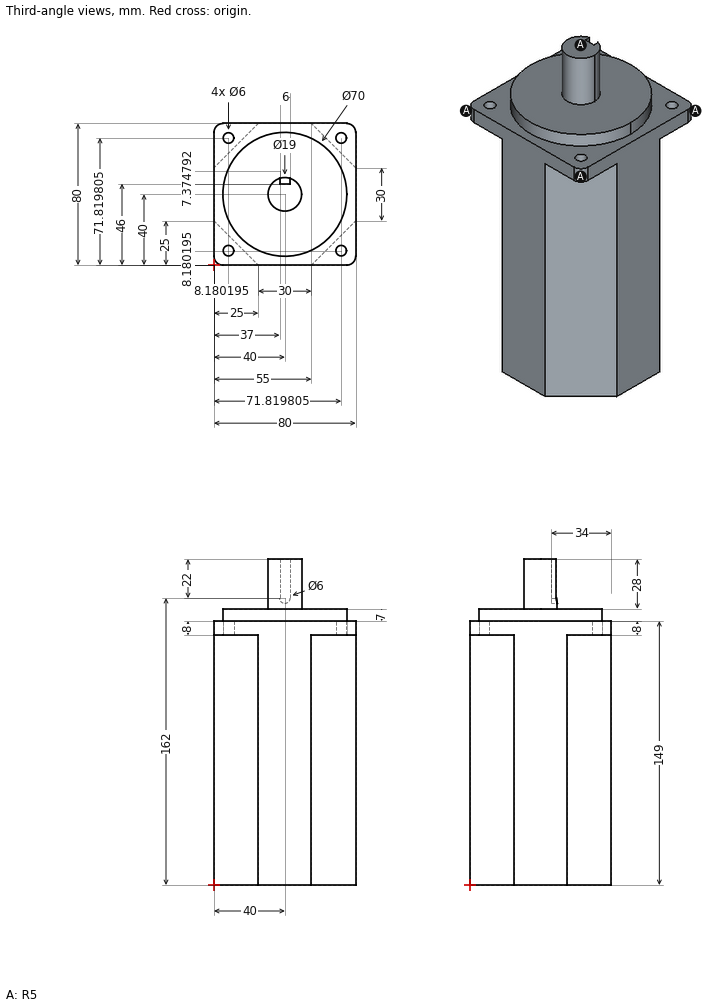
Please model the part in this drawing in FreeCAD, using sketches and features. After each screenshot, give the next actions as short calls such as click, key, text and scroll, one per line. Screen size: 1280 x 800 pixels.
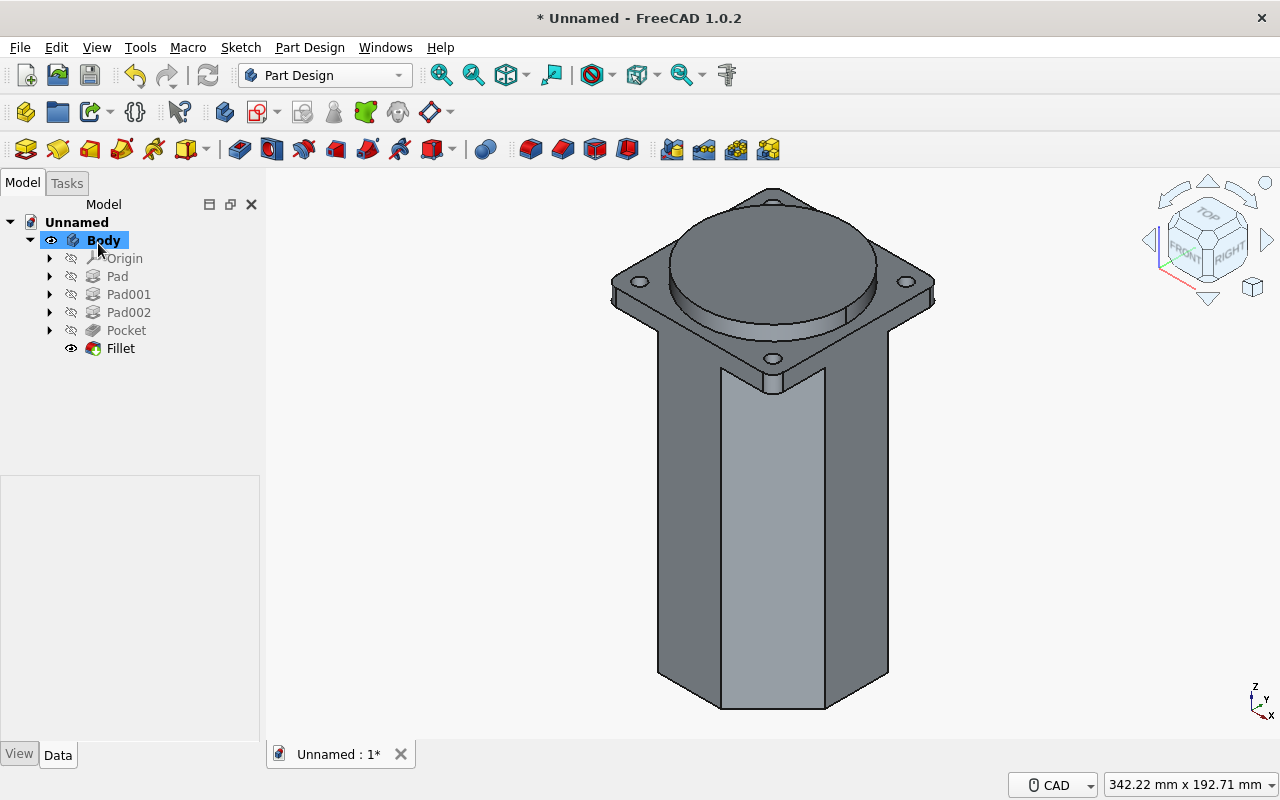
click(442, 76)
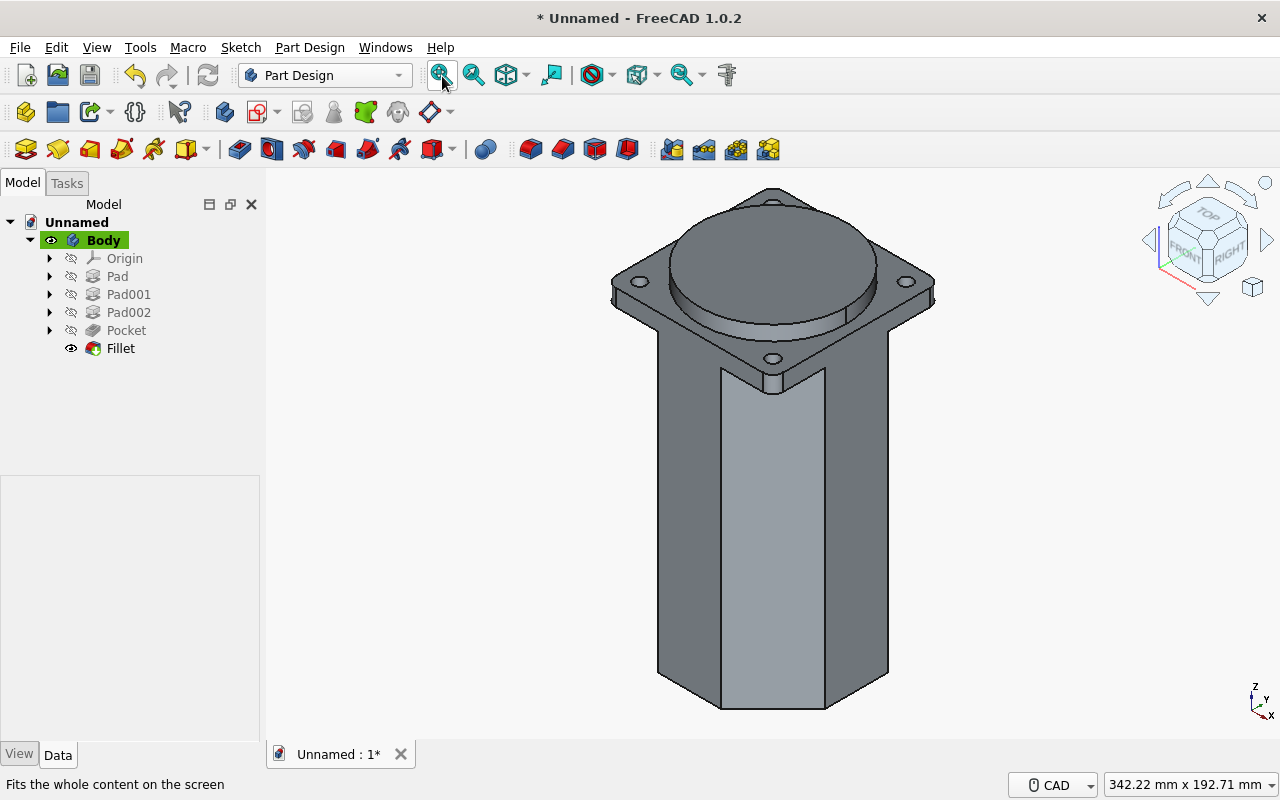
click(773, 264)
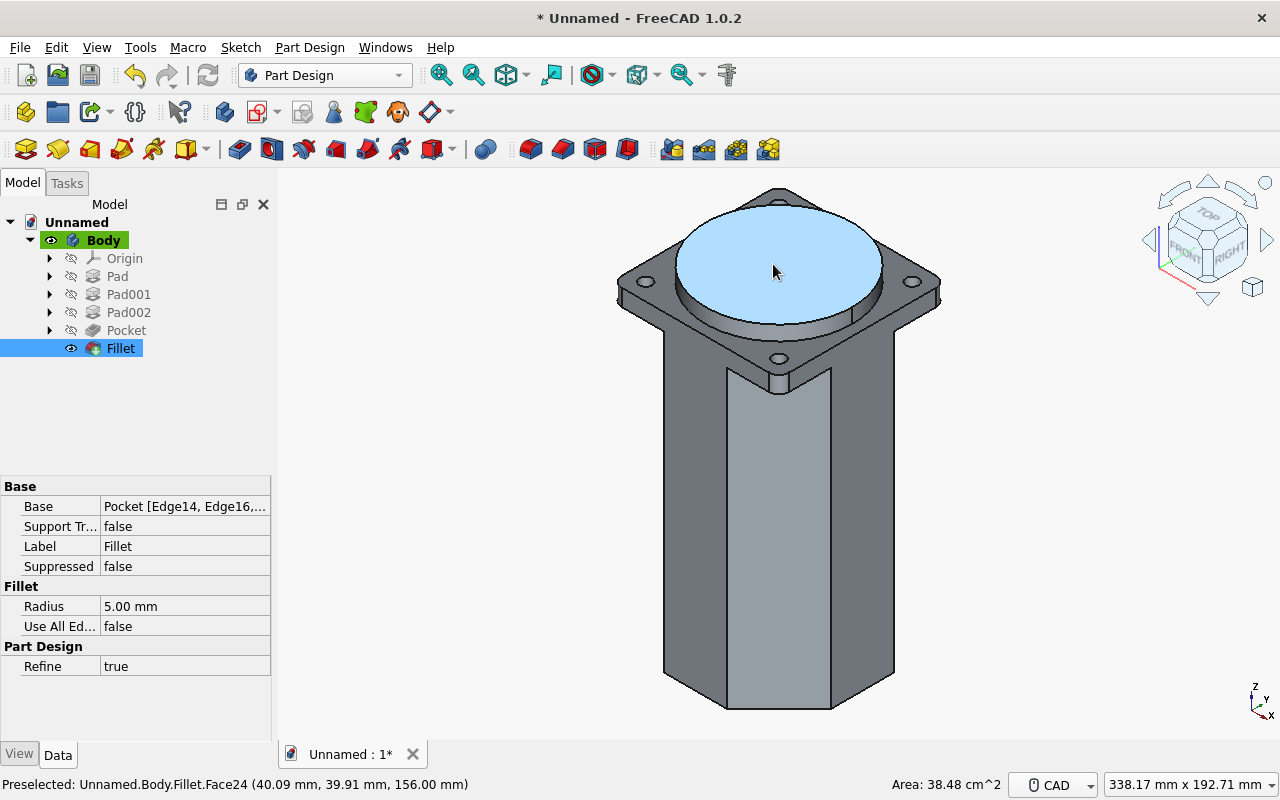
click(258, 112)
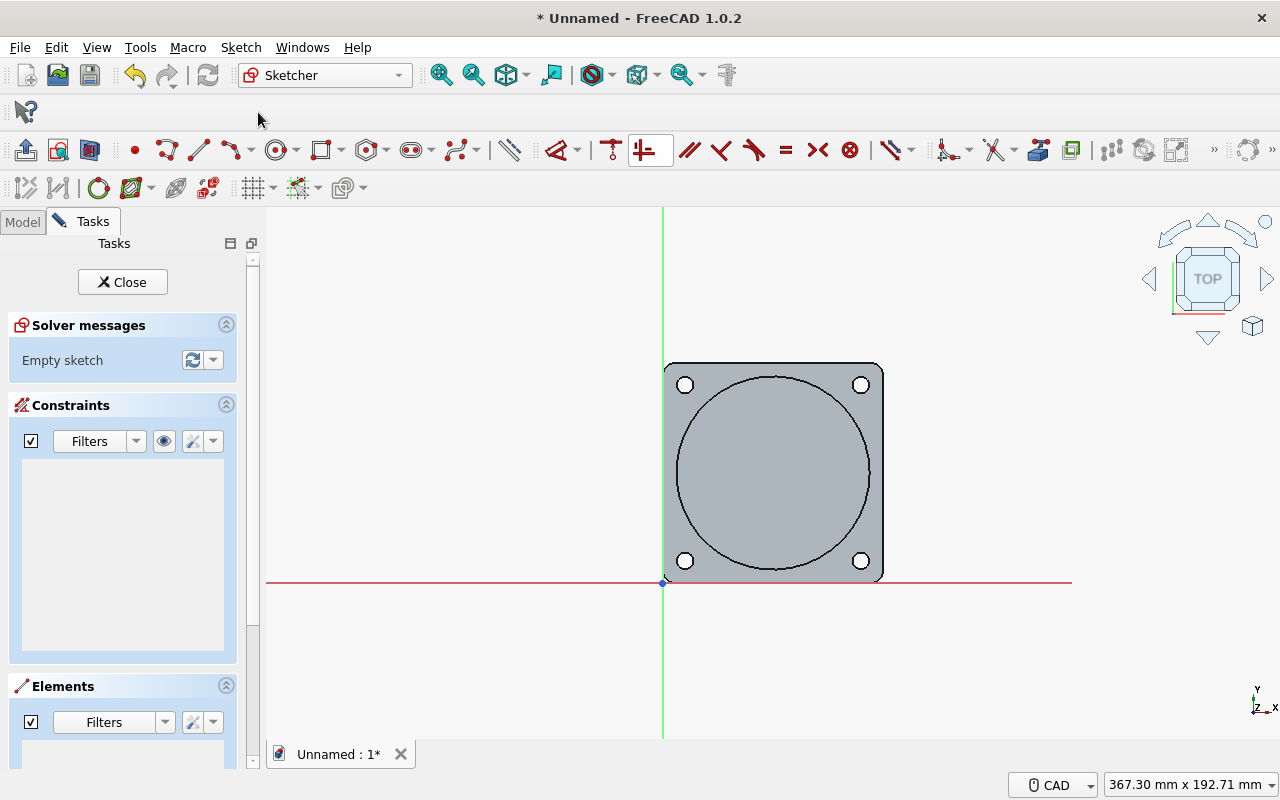
scroll(787, 473, up, 9)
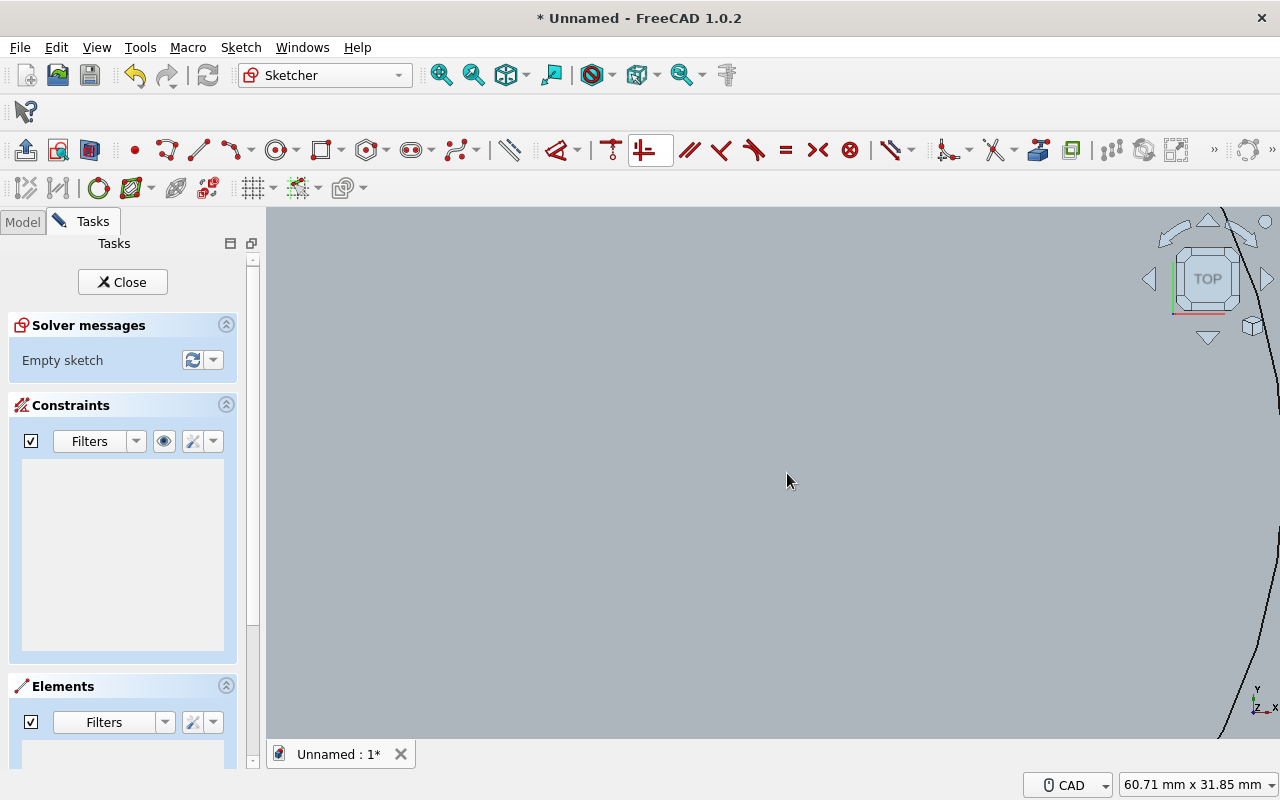
key(g)
key(c)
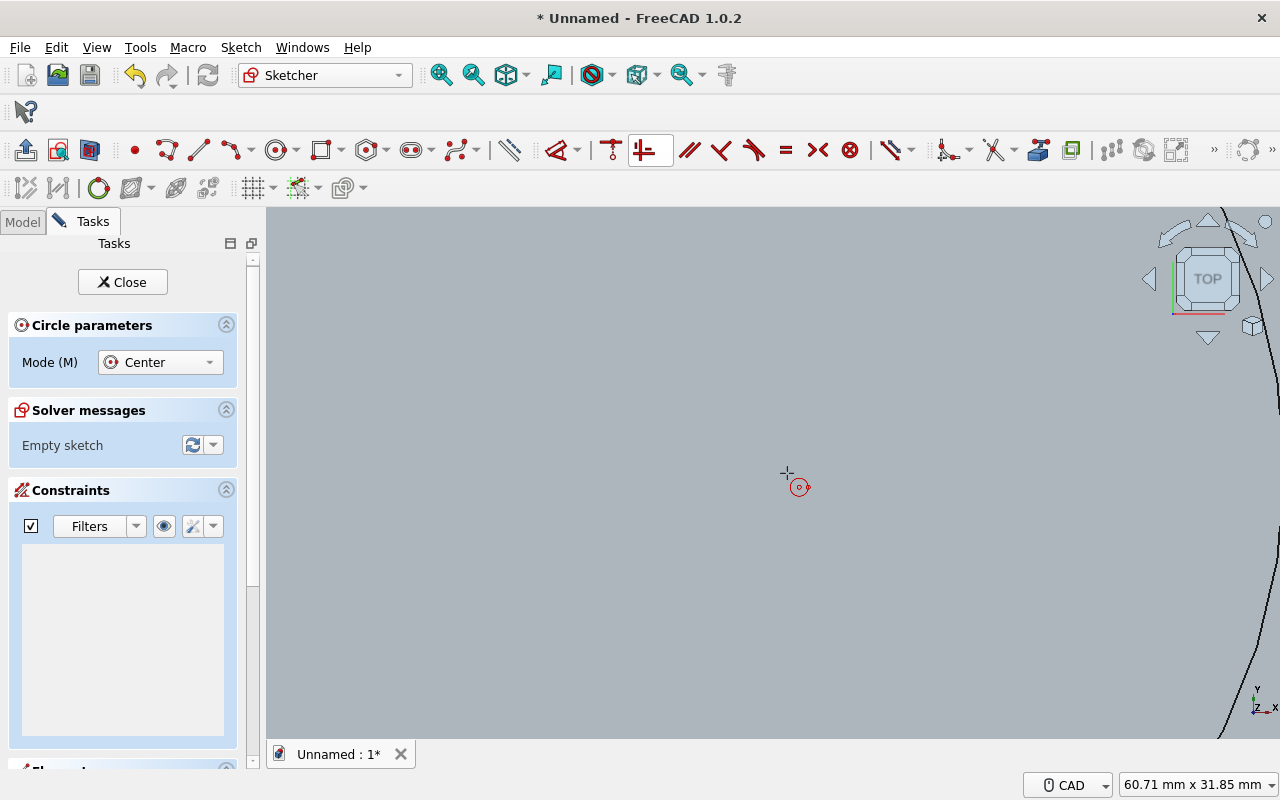
click(700, 470)
click(812, 358)
key(Escape)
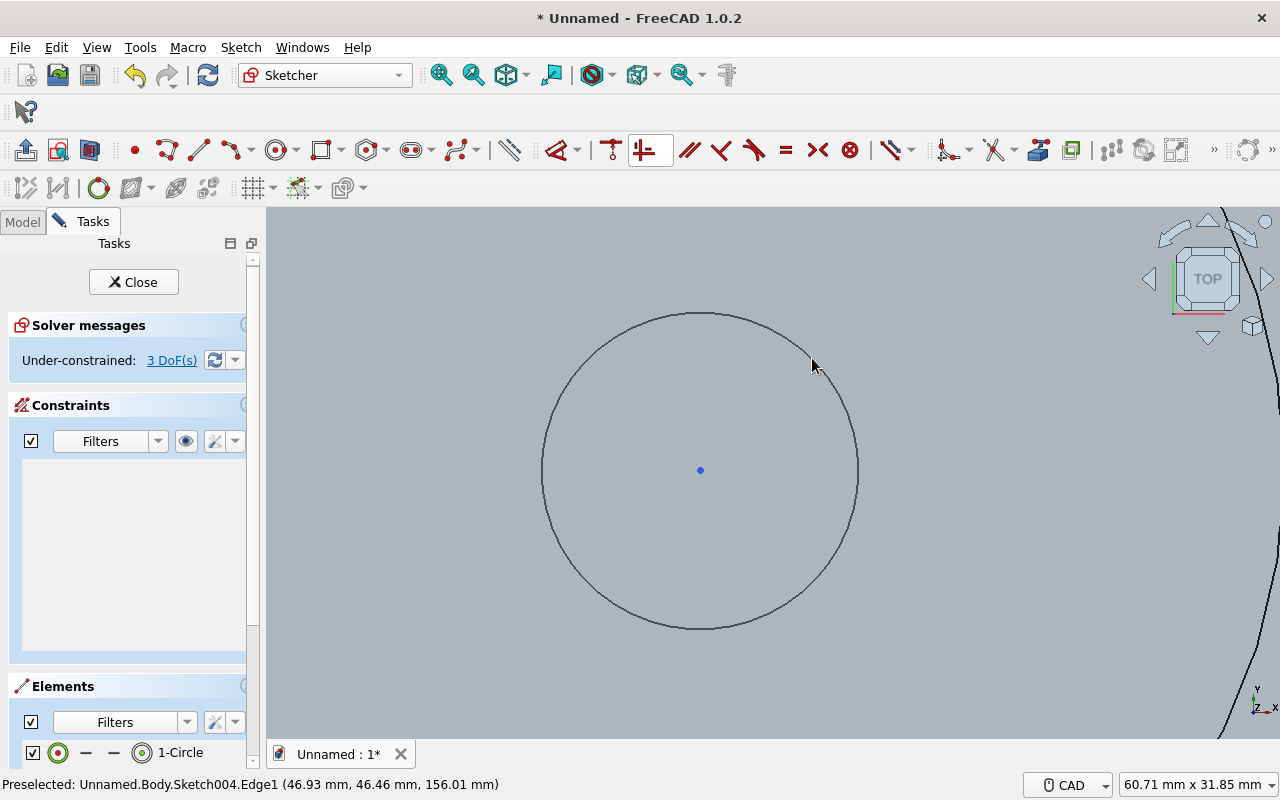
key(d)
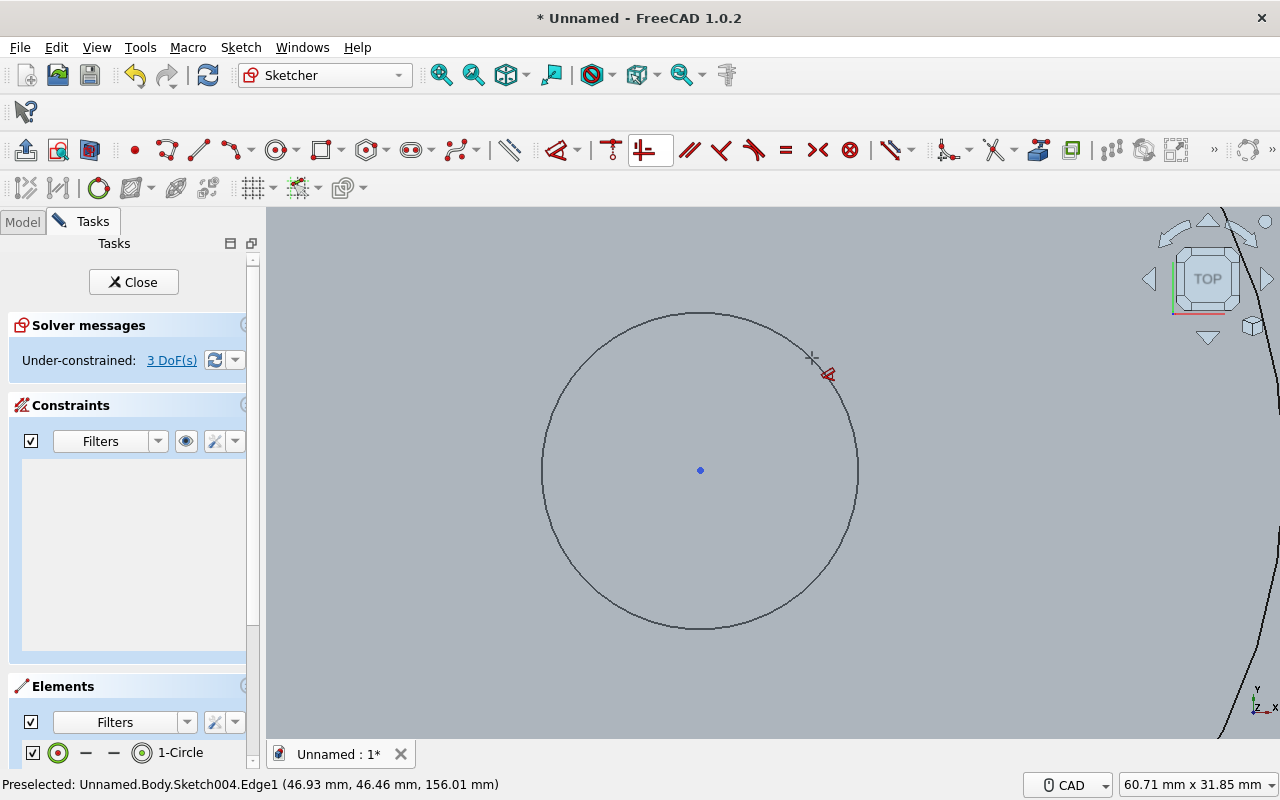
click(812, 359)
click(835, 336)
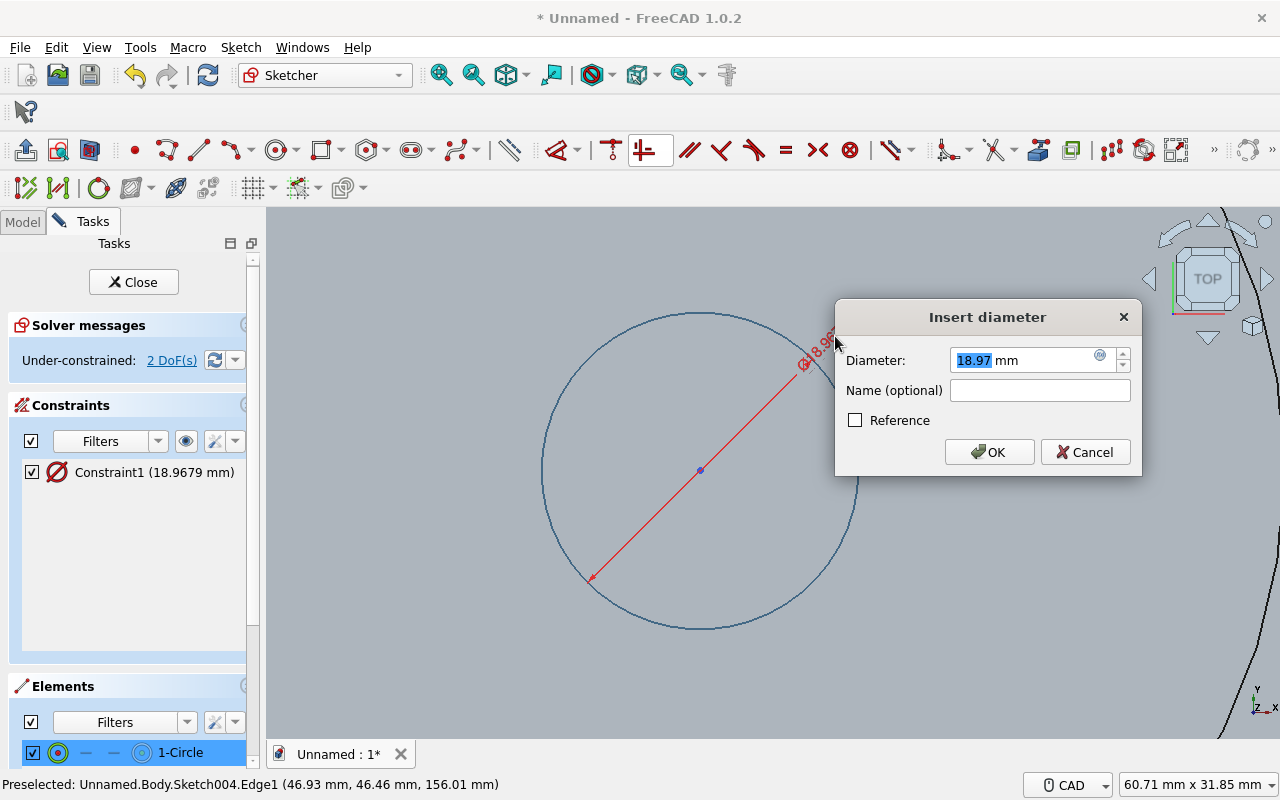
text(19)
key(Return)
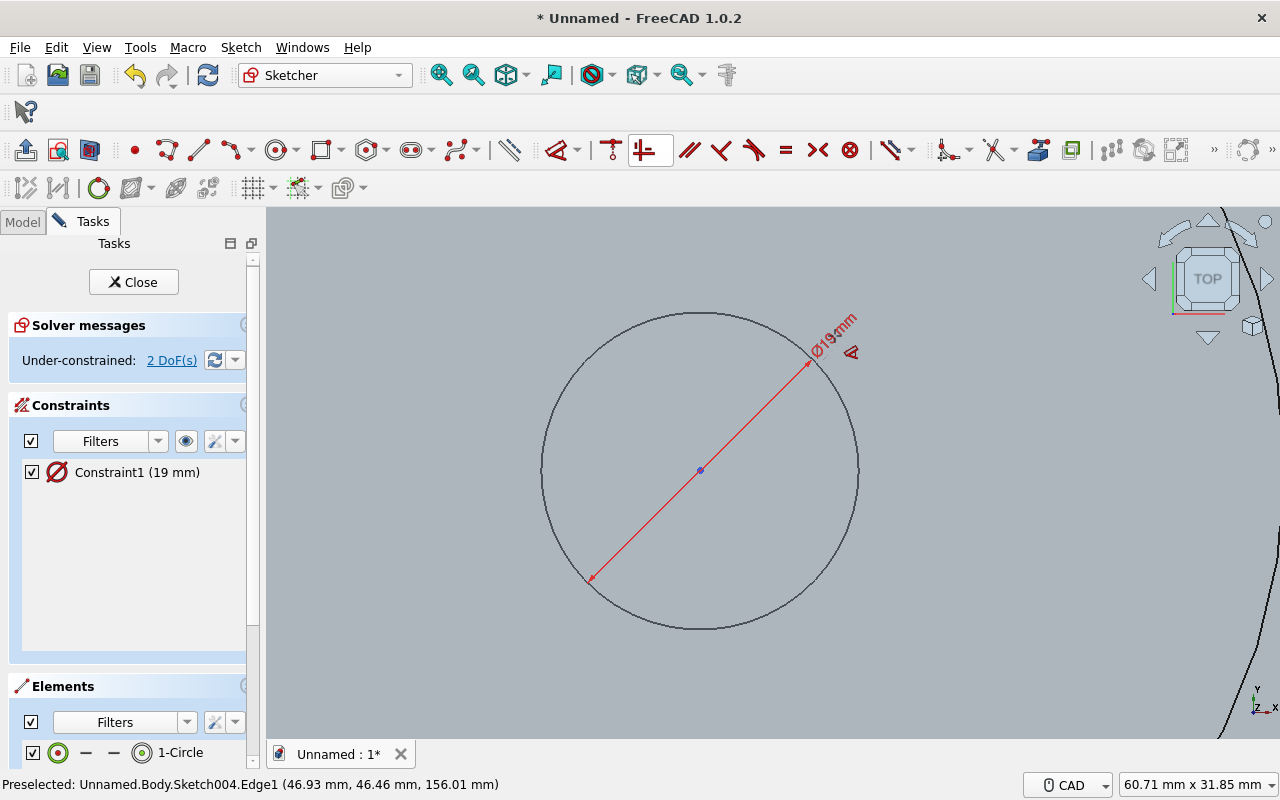
click(700, 471)
click(497, 437)